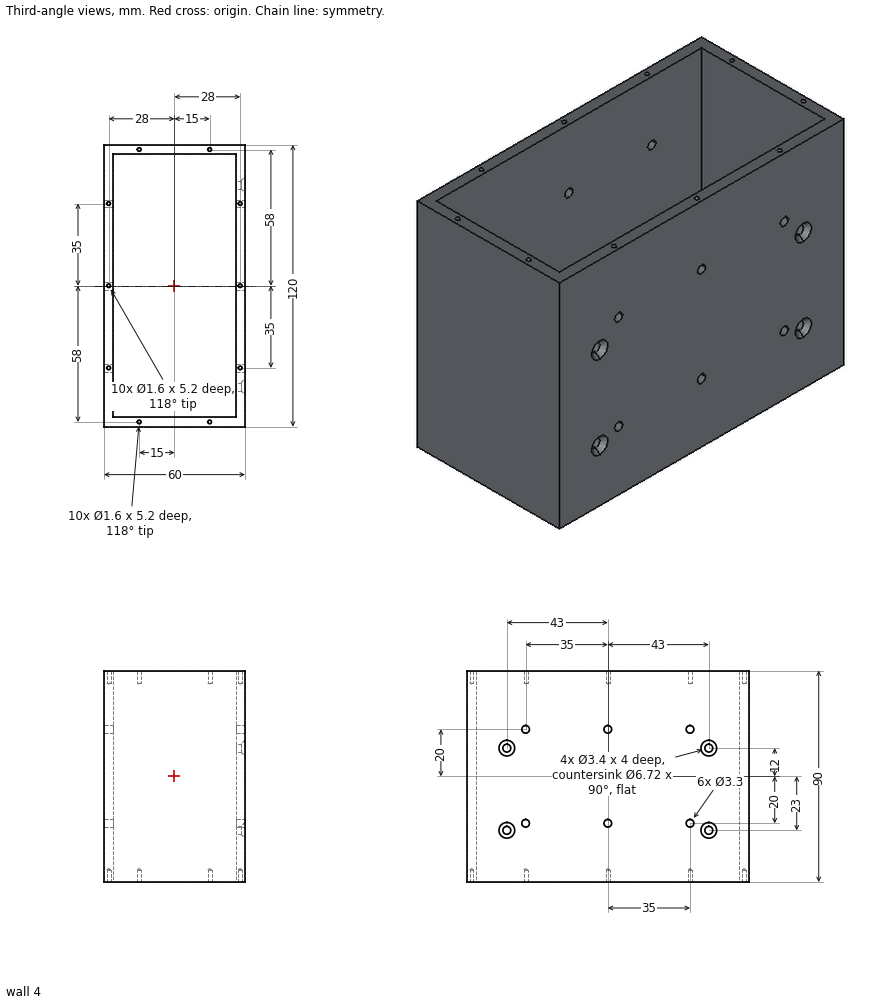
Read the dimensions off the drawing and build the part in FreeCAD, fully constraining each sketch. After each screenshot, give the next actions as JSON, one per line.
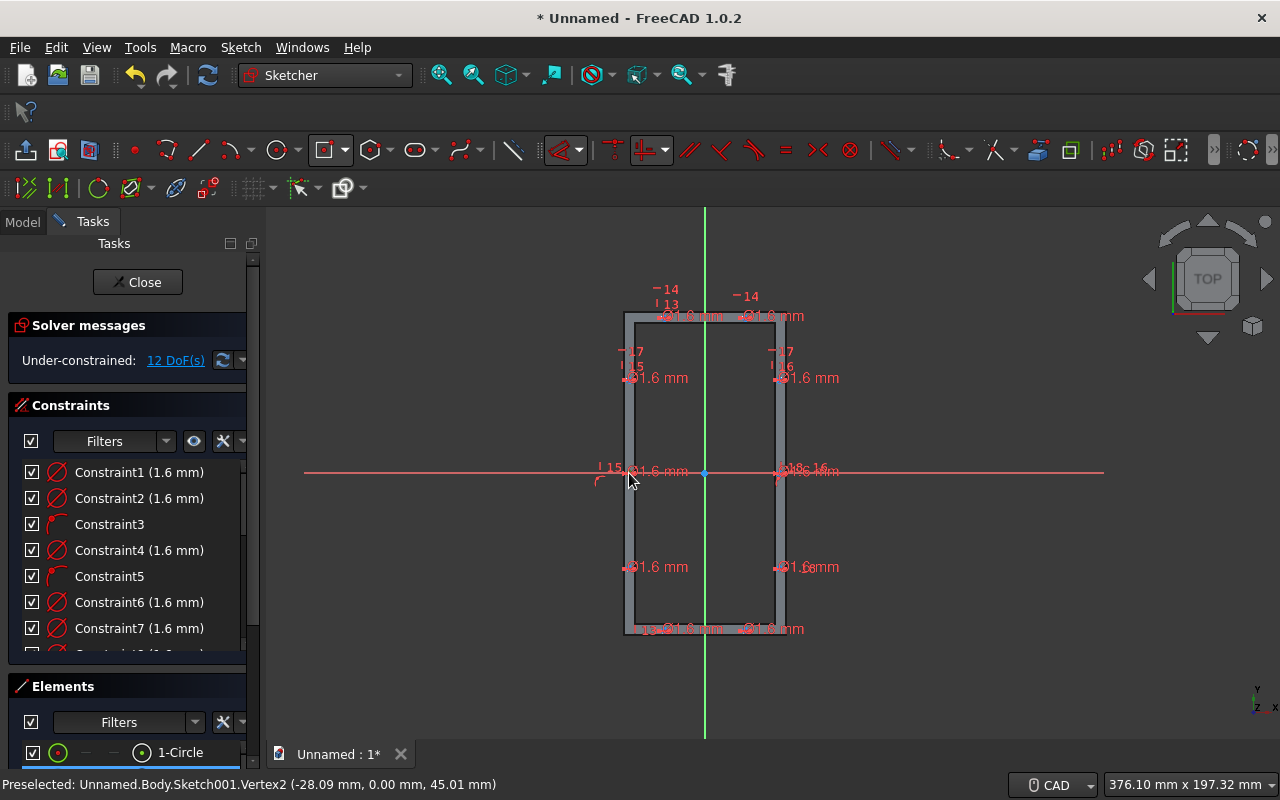
{"action": "left_click", "coordinate": [629, 569]}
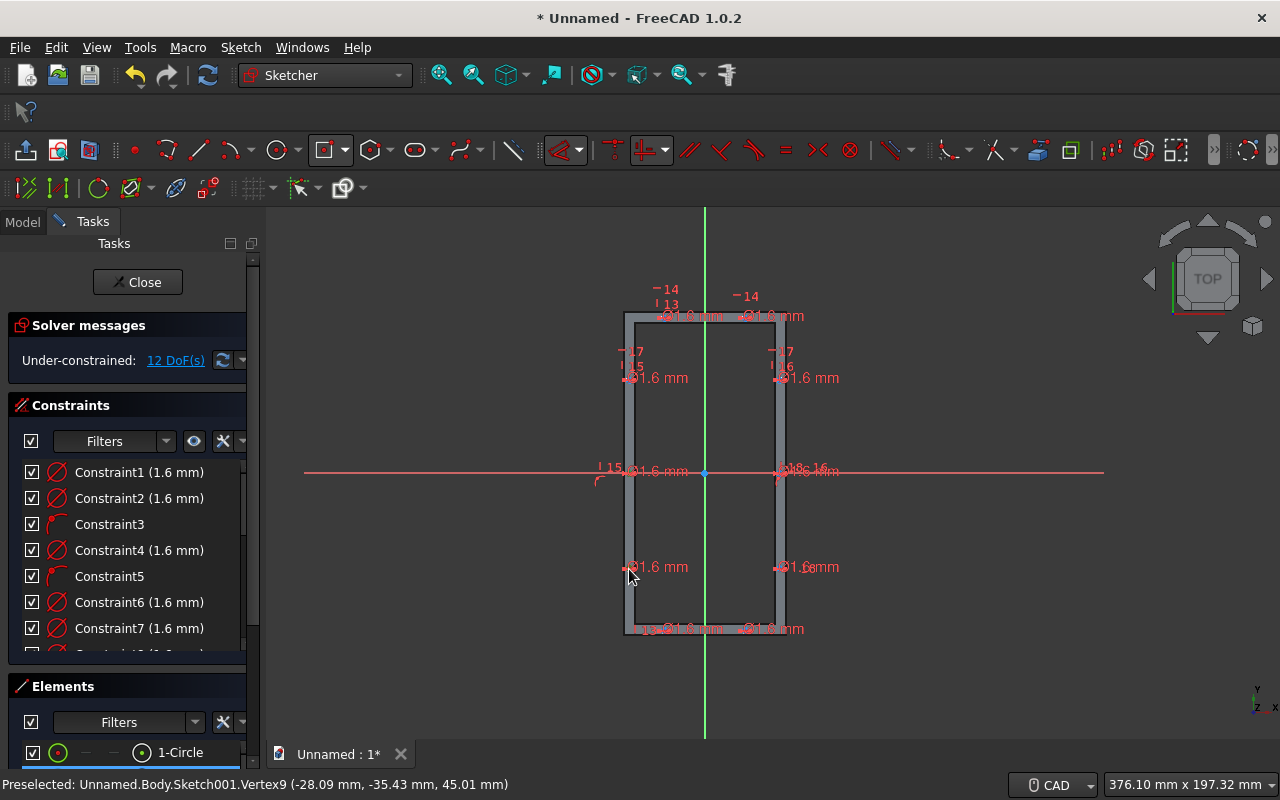
{"action": "left_click", "coordinate": [668, 150]}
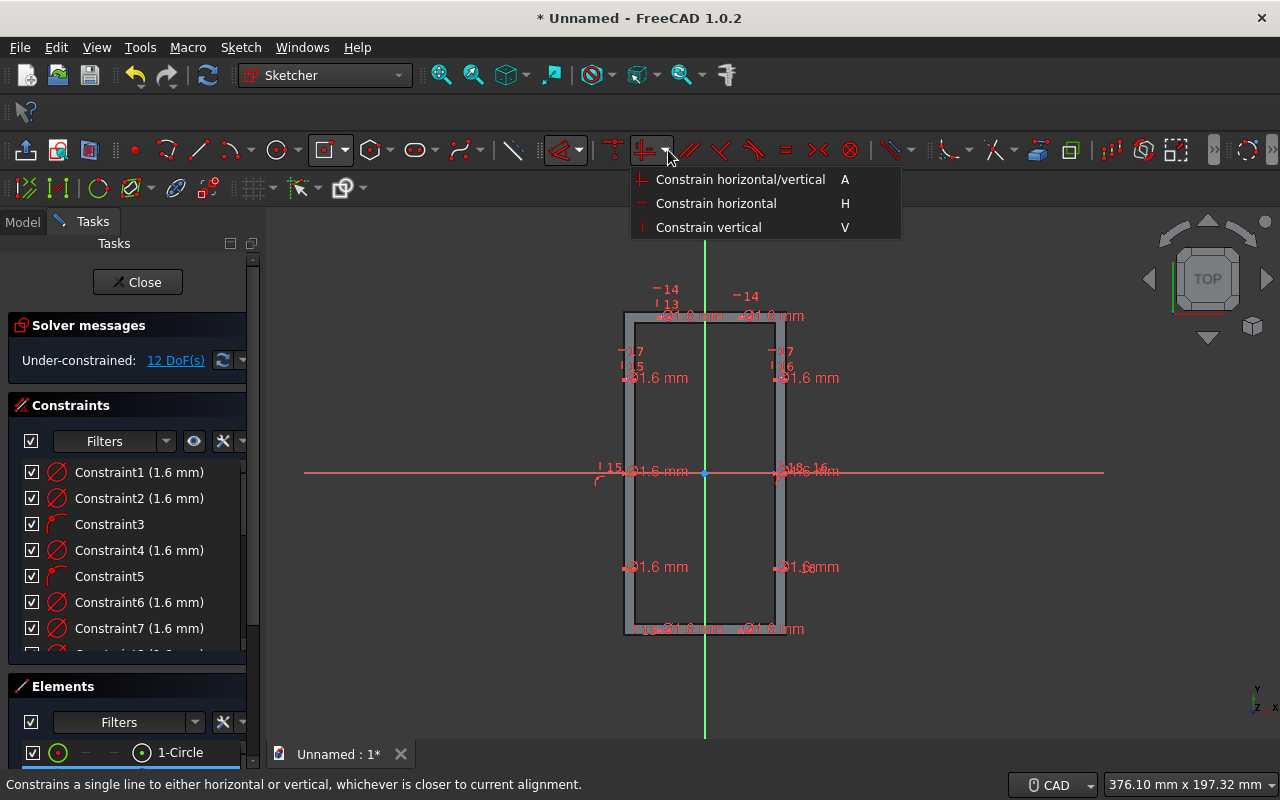
{"action": "left_click", "coordinate": [766, 227]}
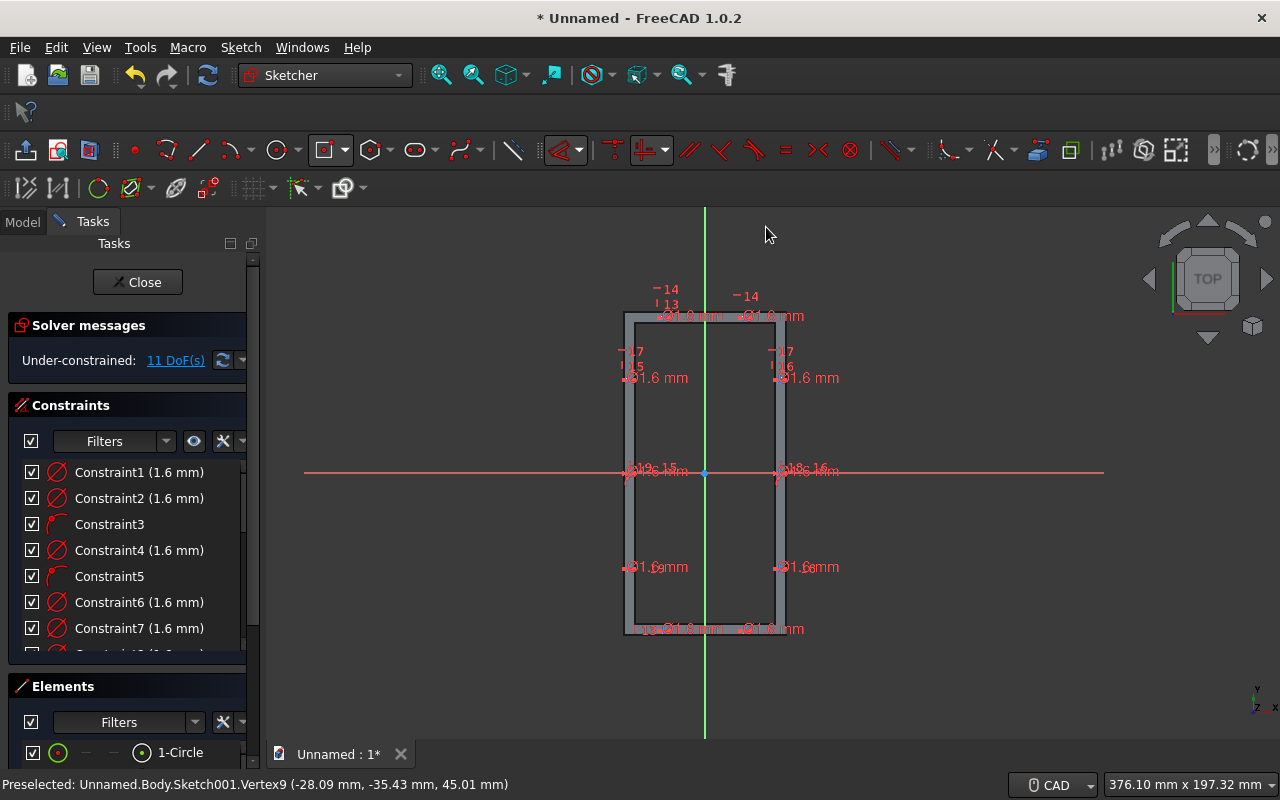
{"action": "left_click", "coordinate": [780, 569]}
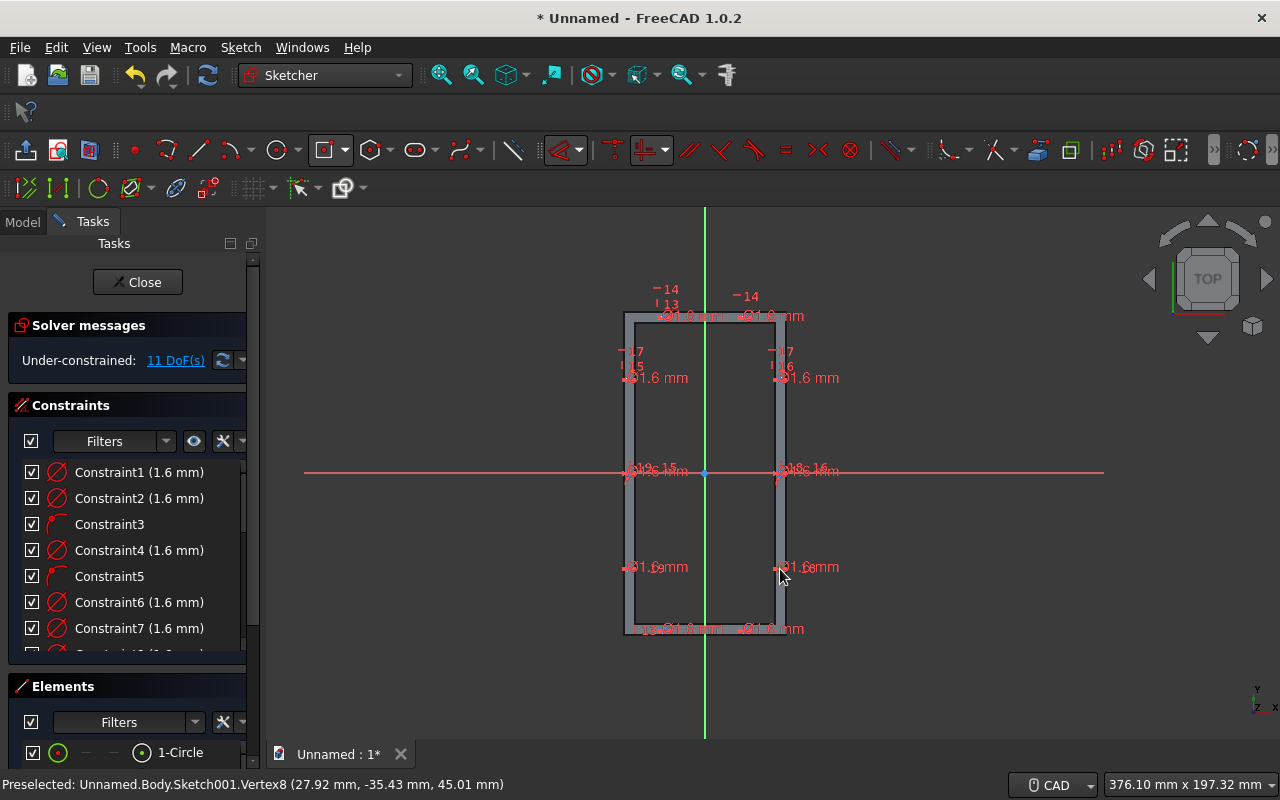
{"action": "left_click", "coordinate": [629, 569]}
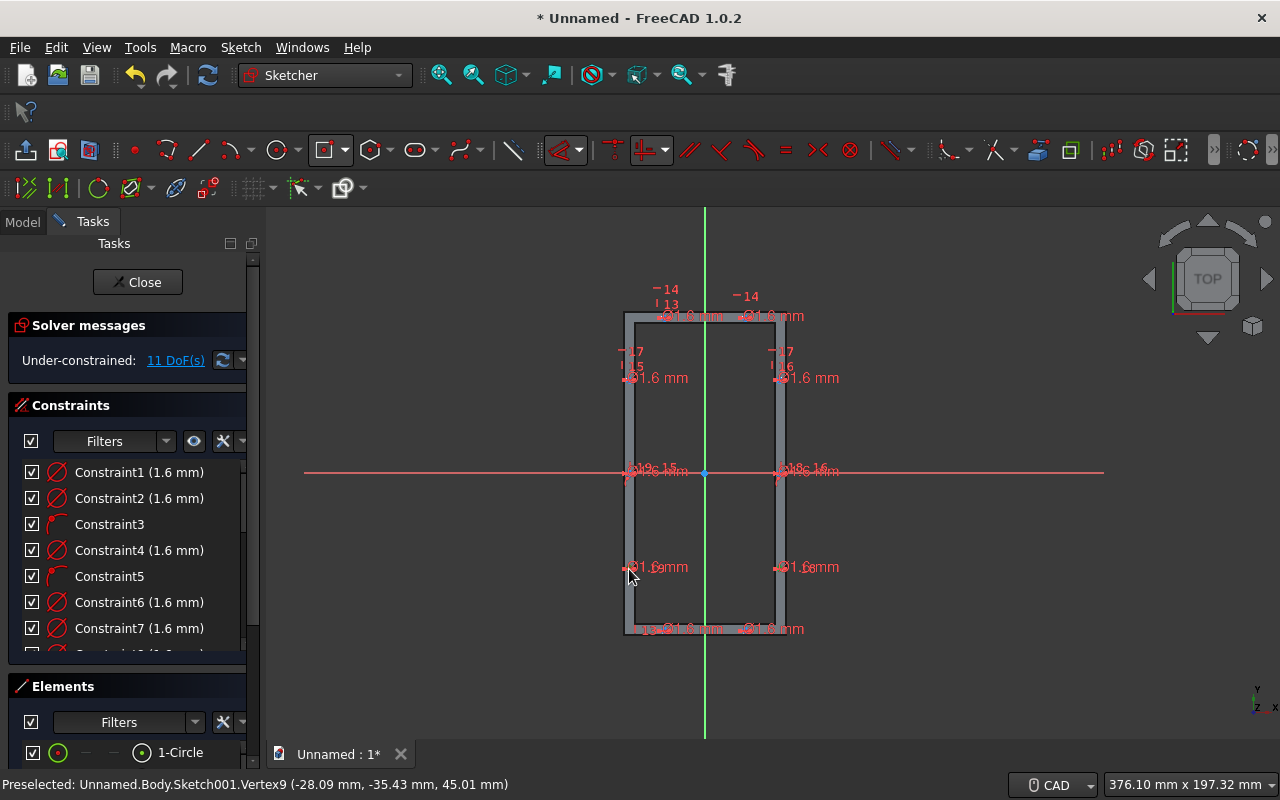
{"action": "key", "text": "h"}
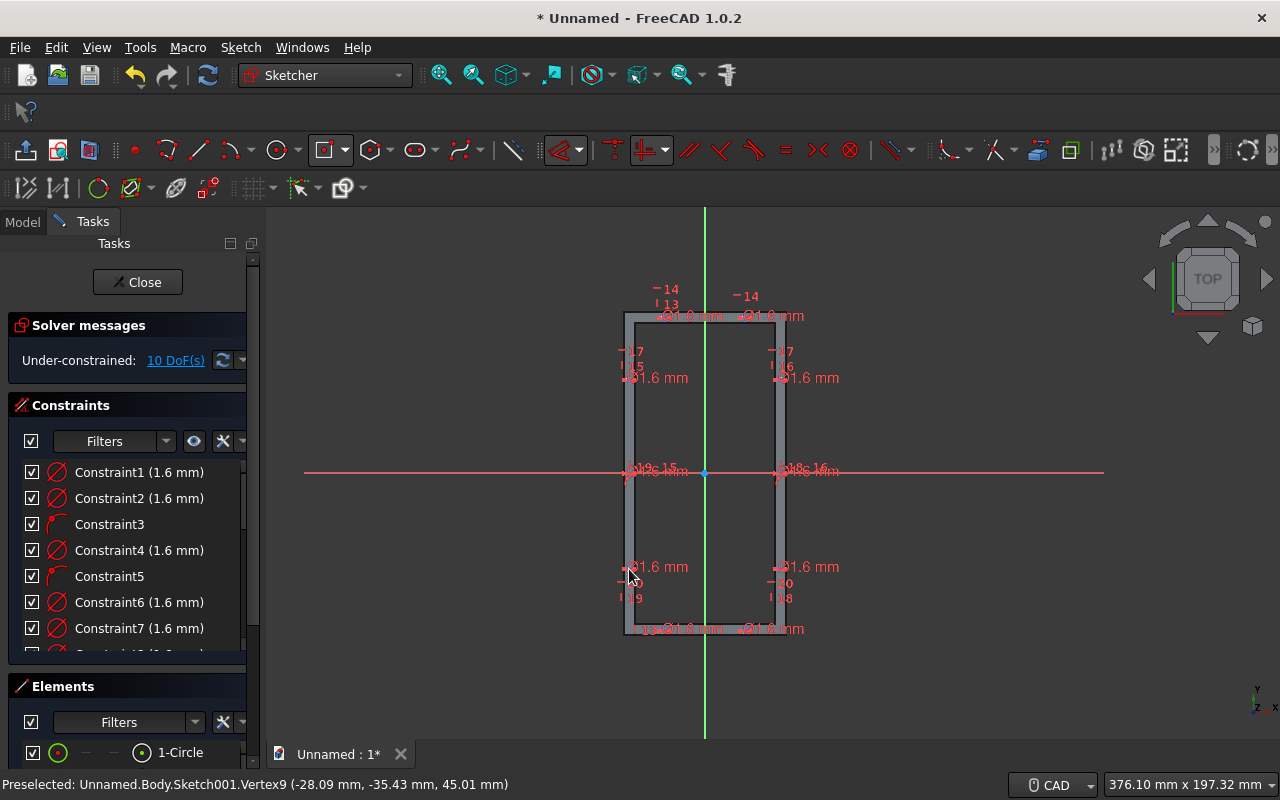
{"action": "left_click", "coordinate": [664, 631]}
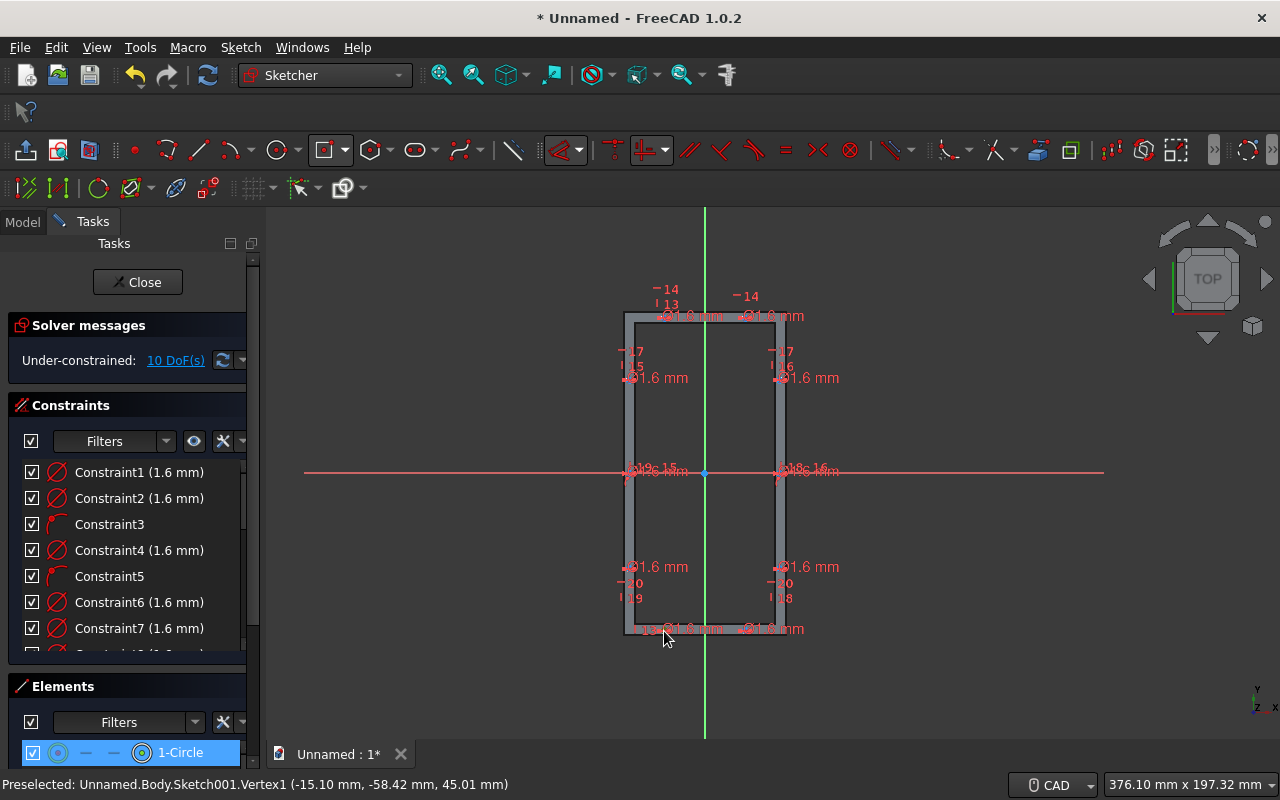
{"action": "left_click", "coordinate": [745, 631]}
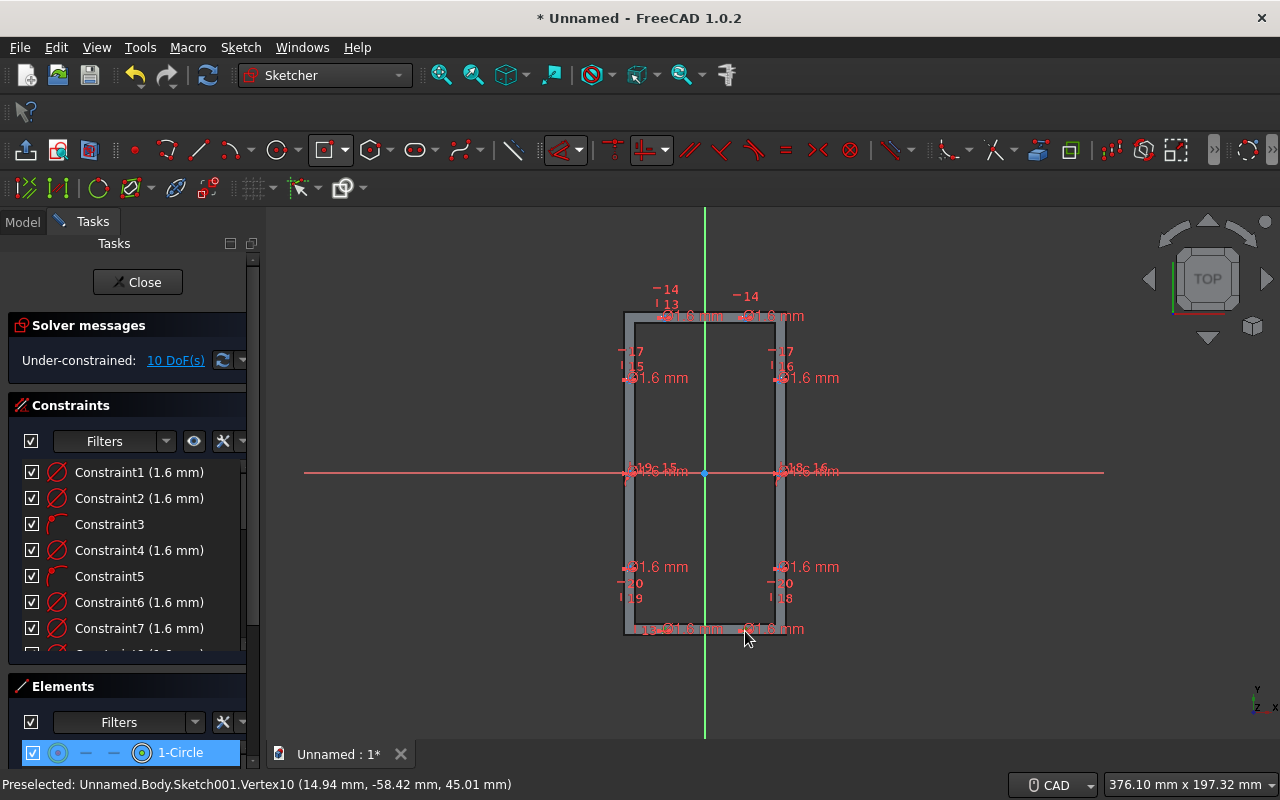
{"action": "left_click", "coordinate": [668, 150]}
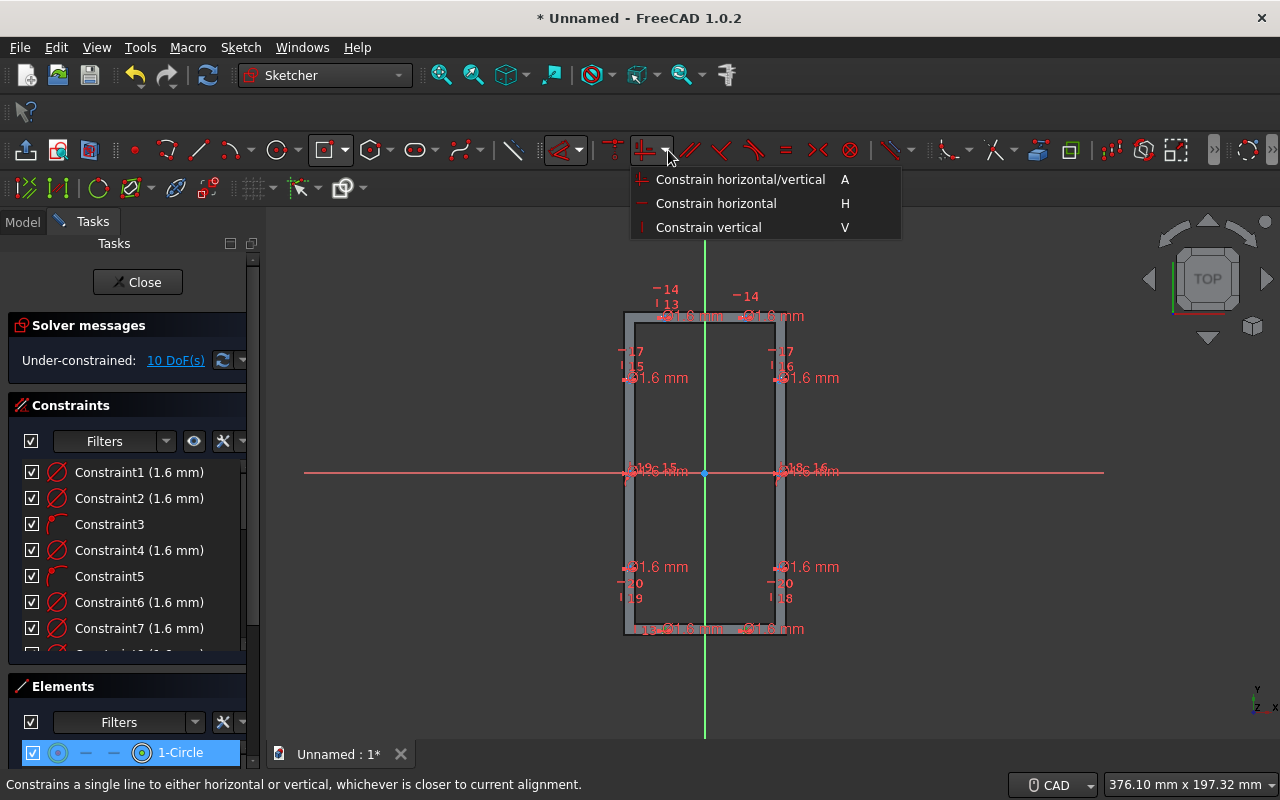
{"action": "left_click", "coordinate": [766, 203]}